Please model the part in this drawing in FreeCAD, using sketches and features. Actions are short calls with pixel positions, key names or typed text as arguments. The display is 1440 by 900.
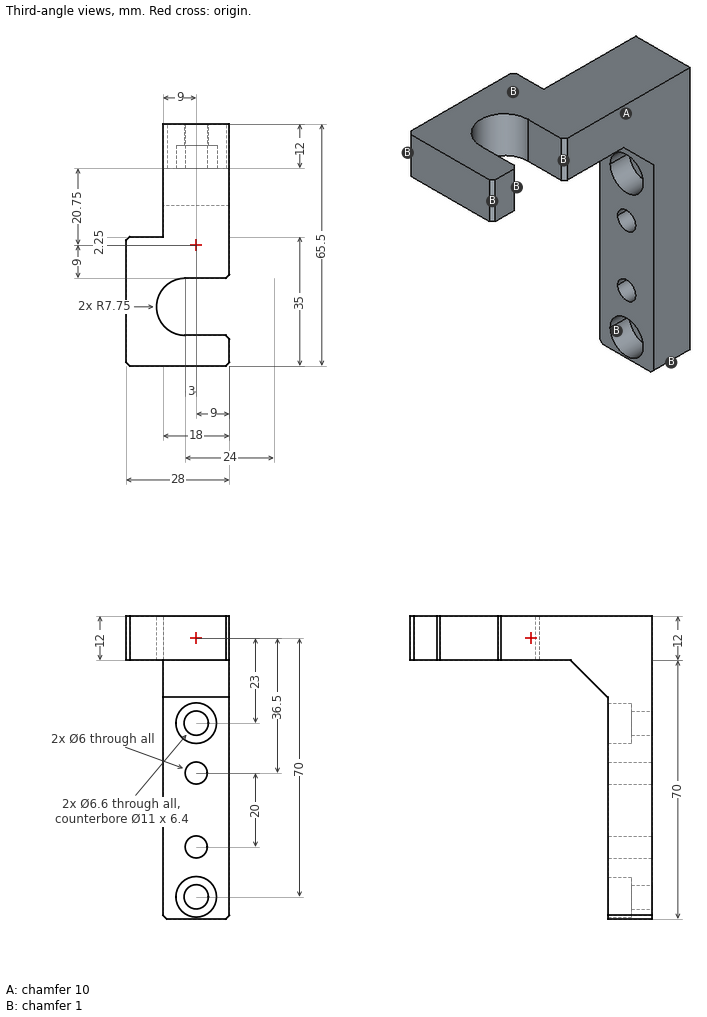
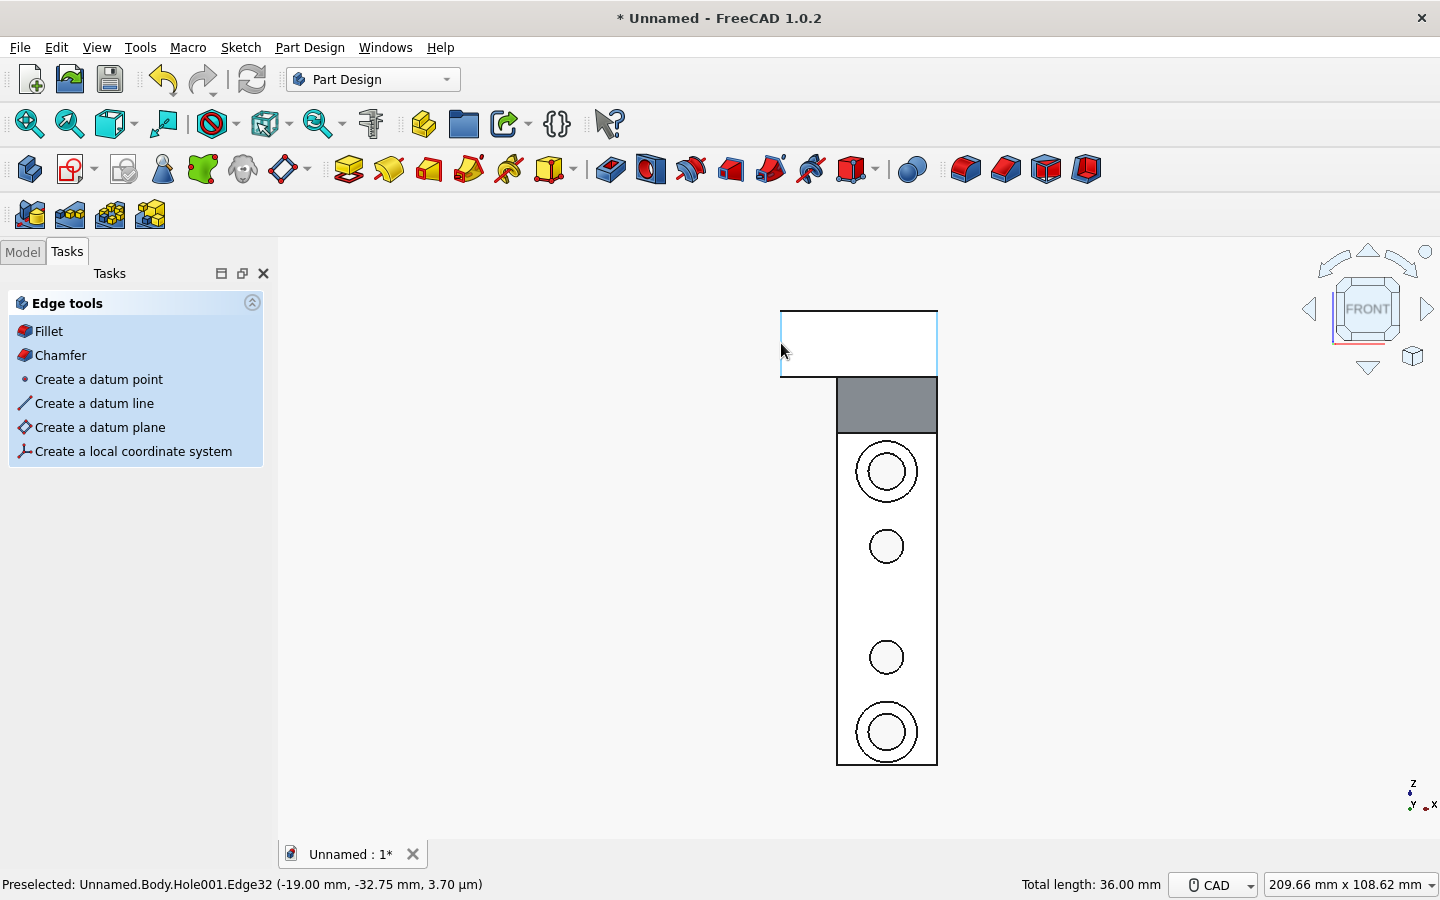
key(3)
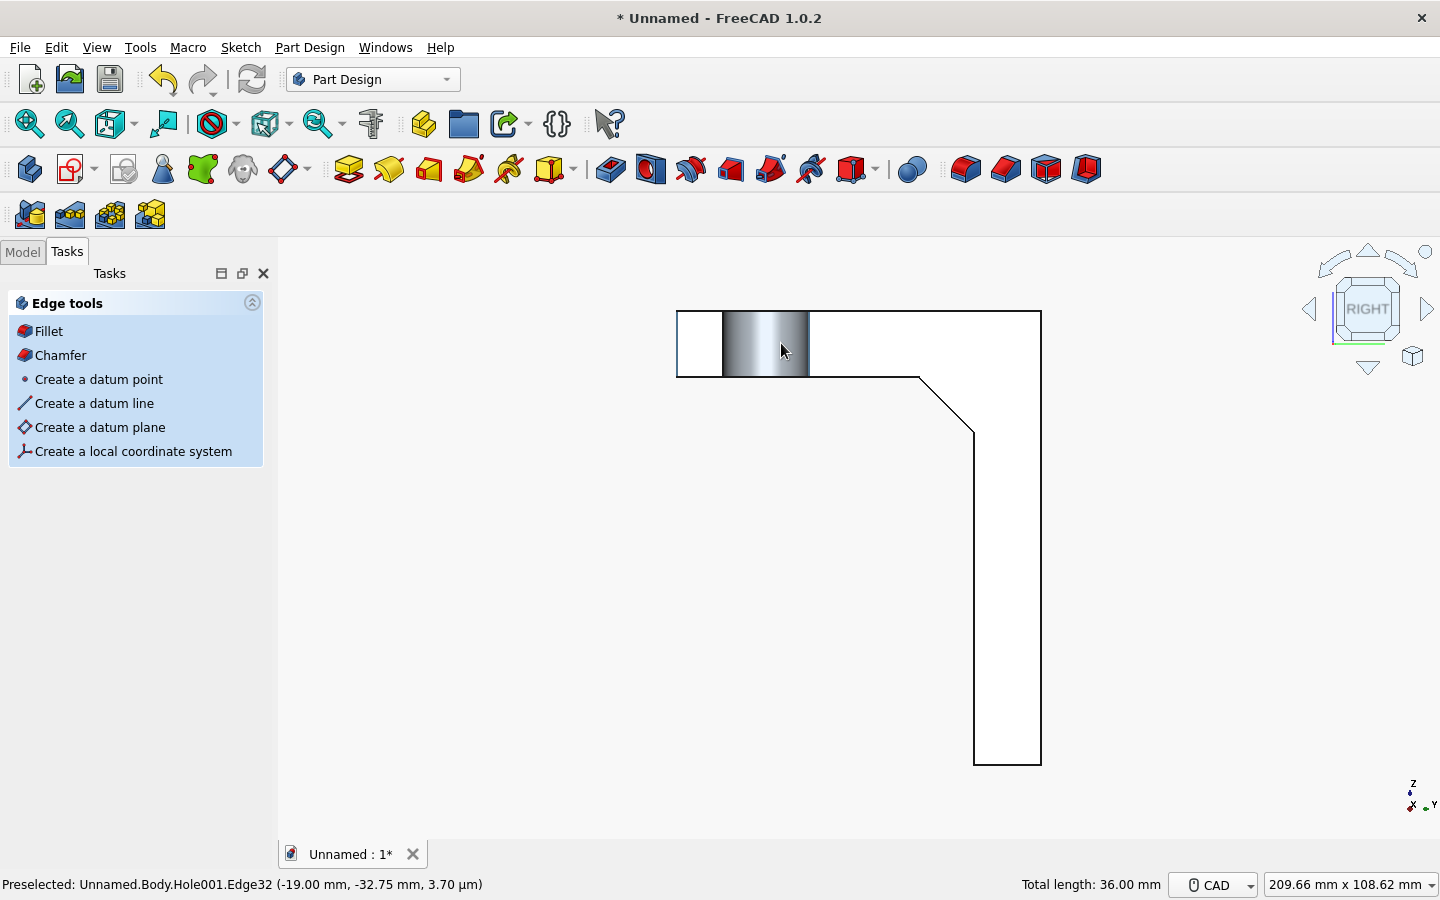
click(723, 343, ctrl)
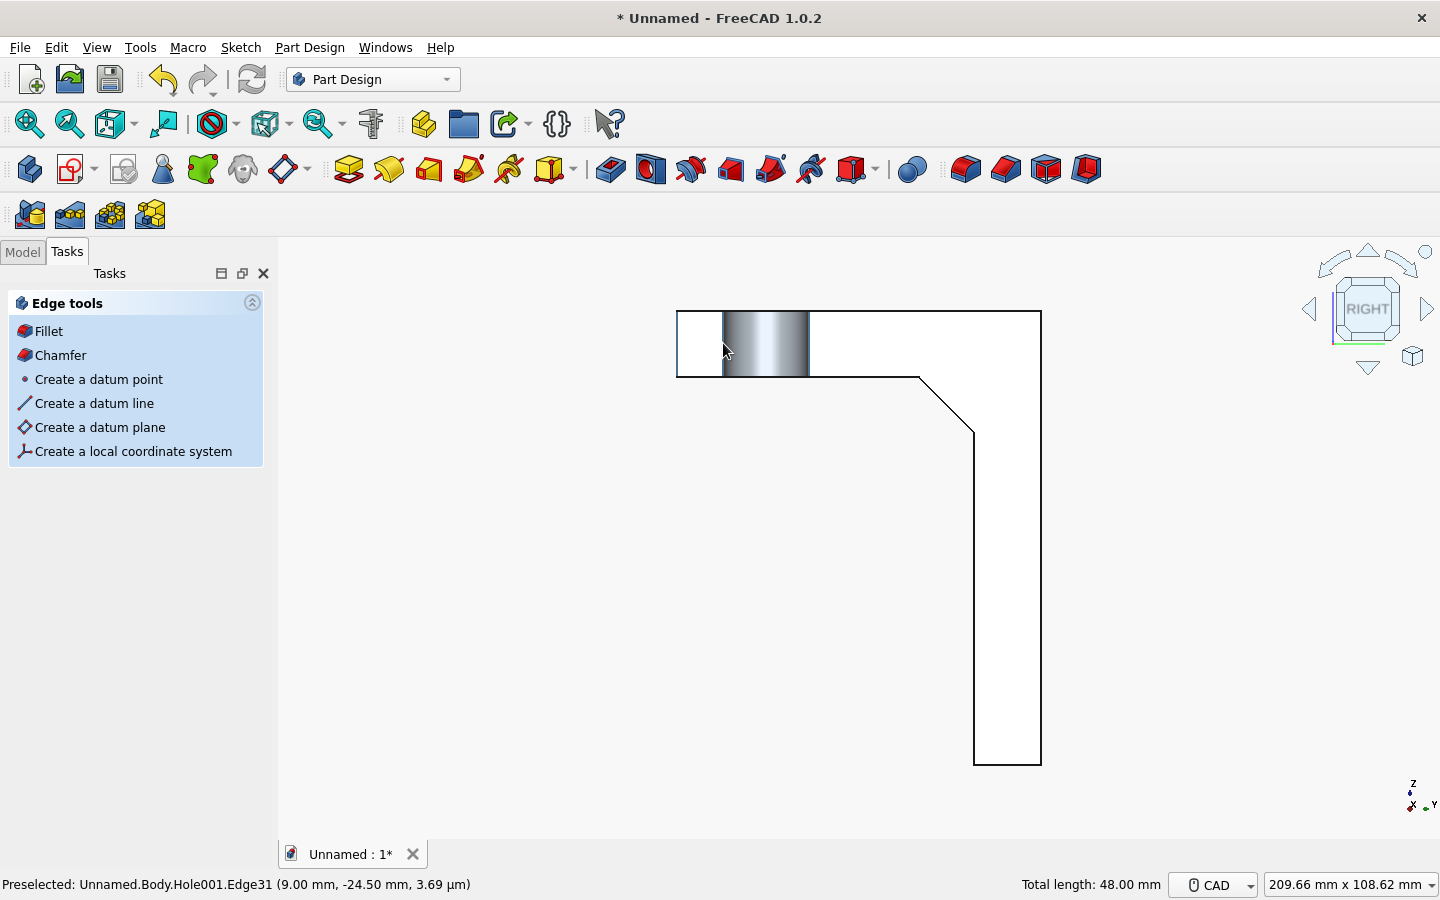
click(1007, 764, ctrl)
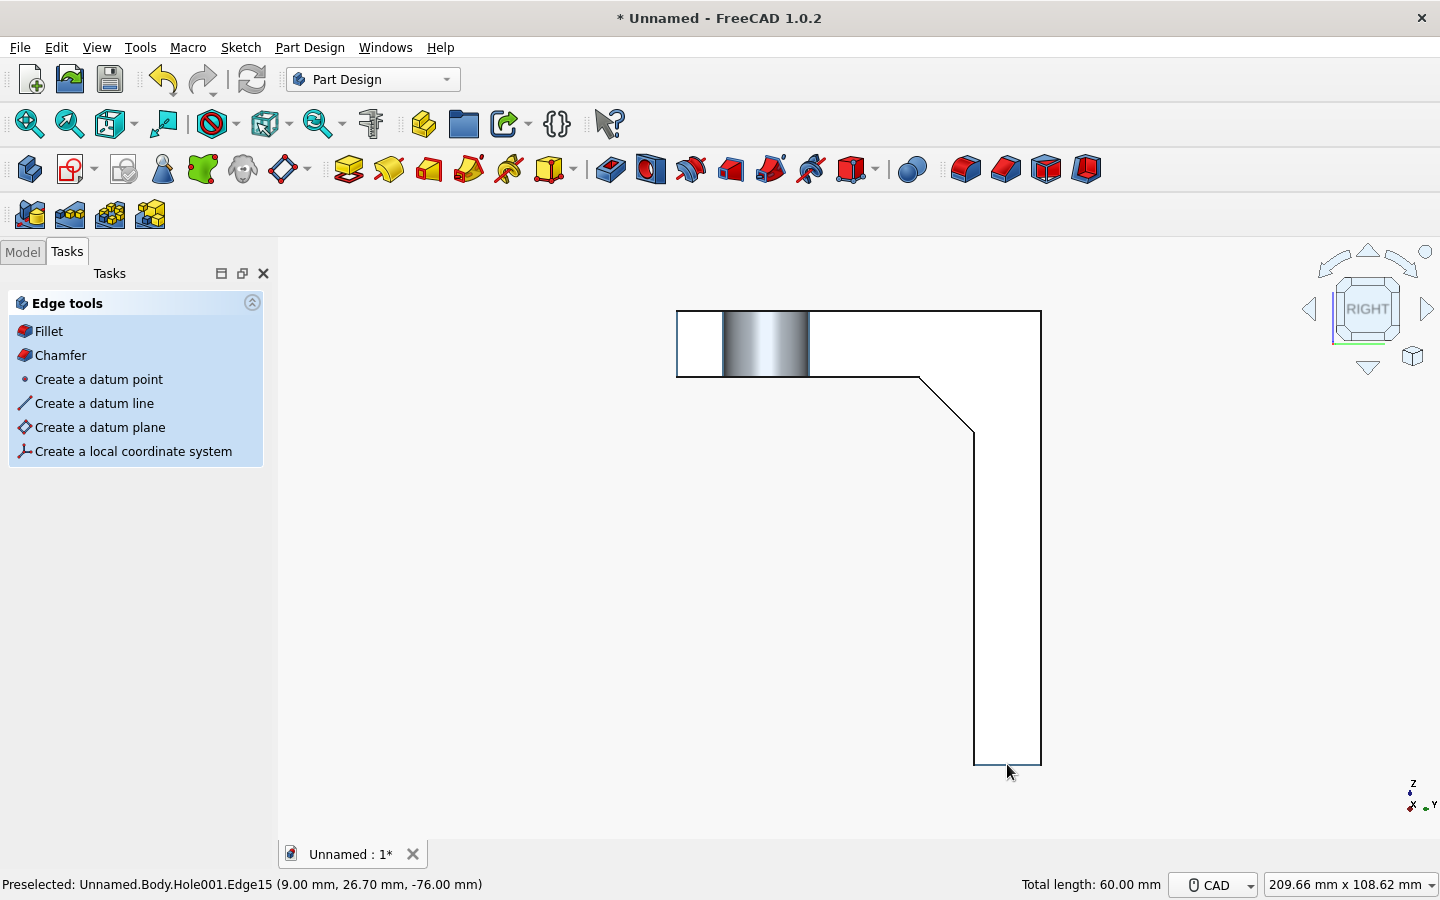
key(5)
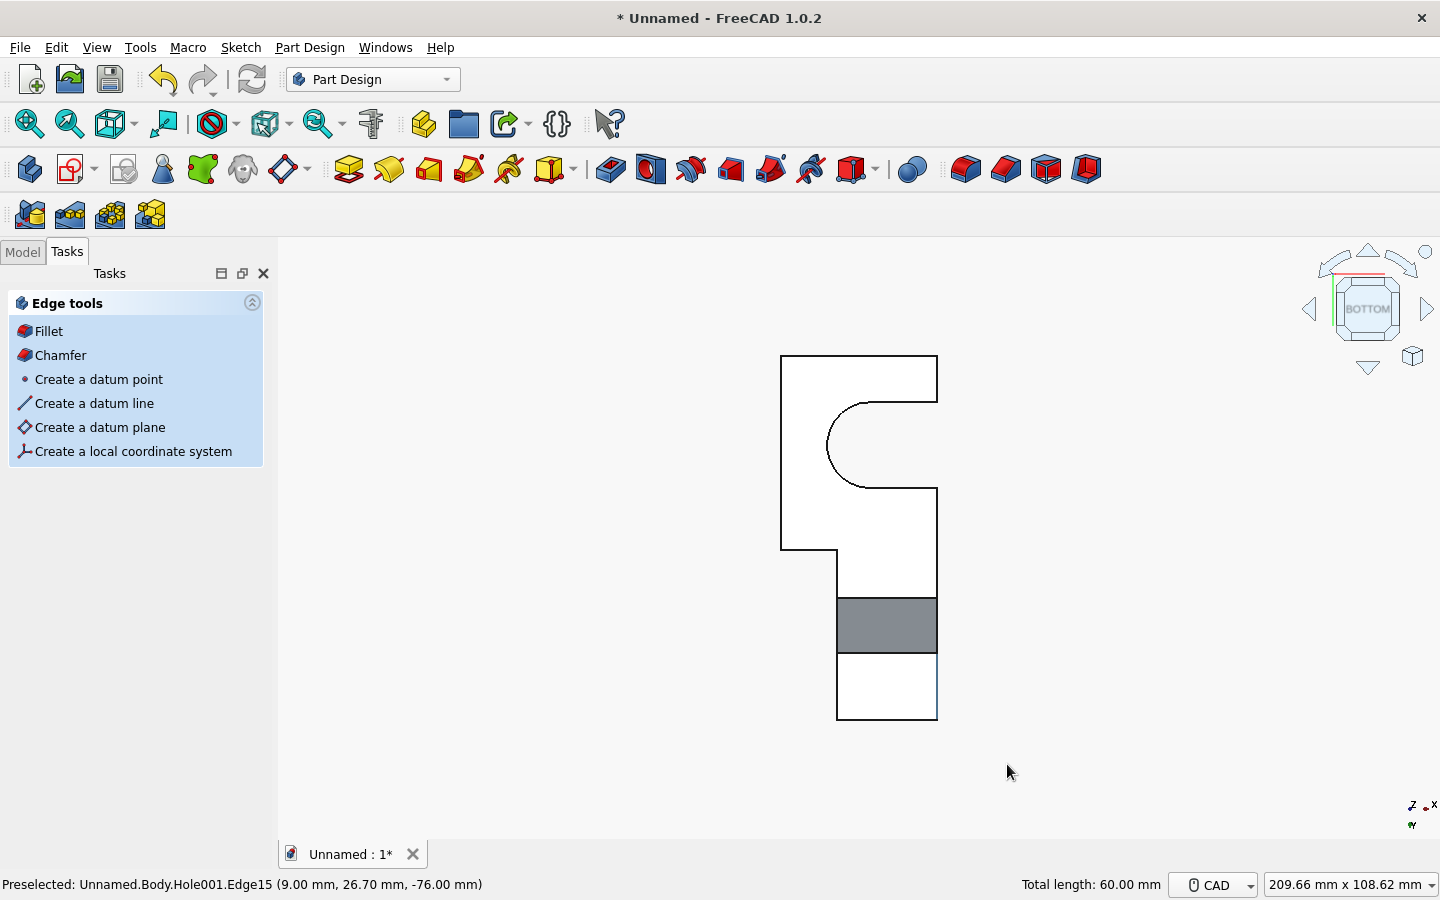
click(837, 685, ctrl)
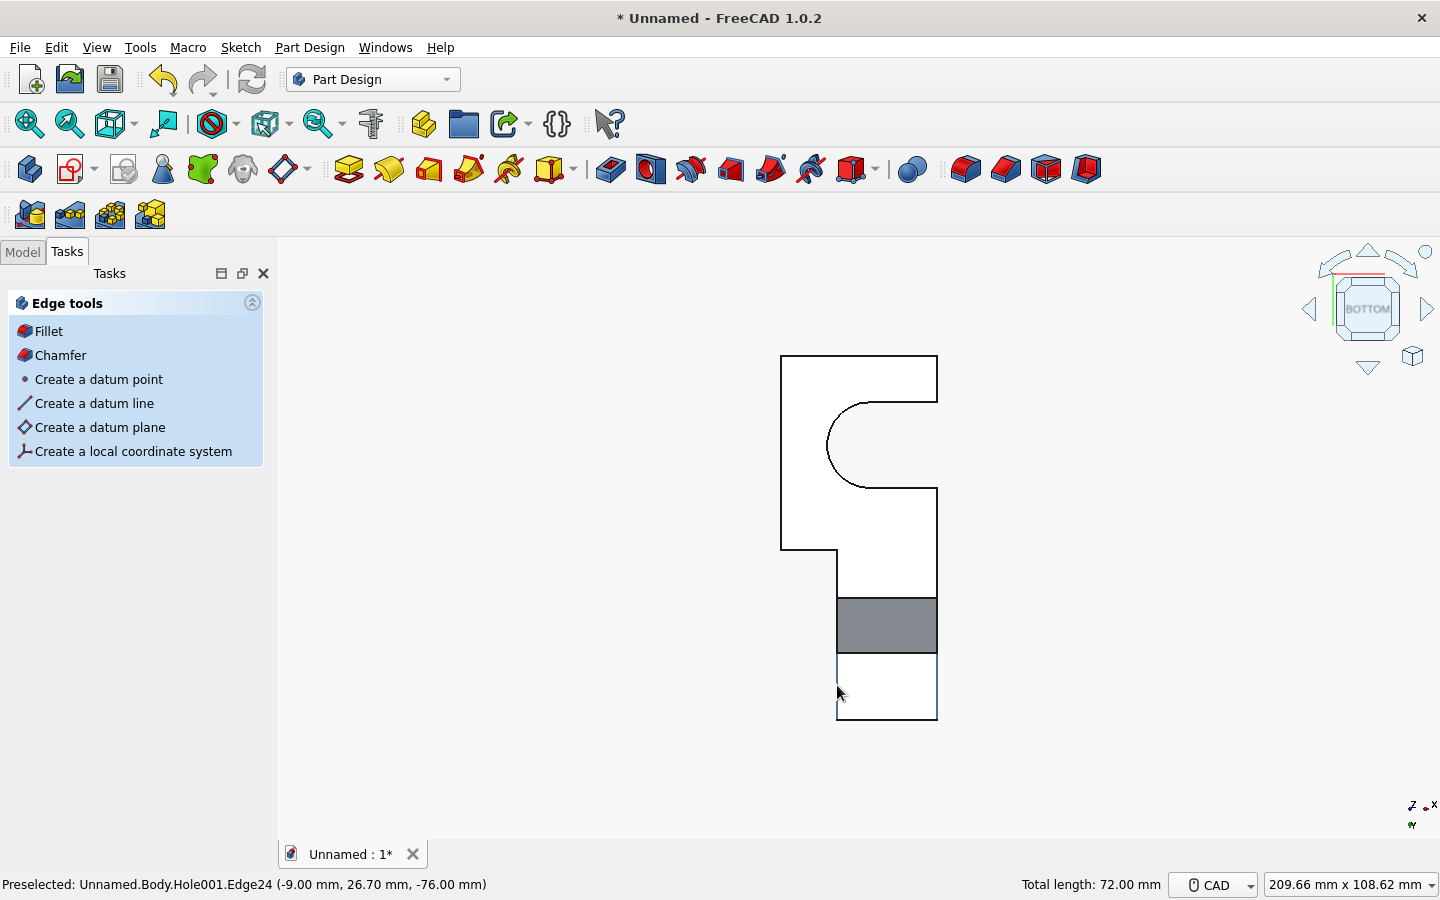
key(4)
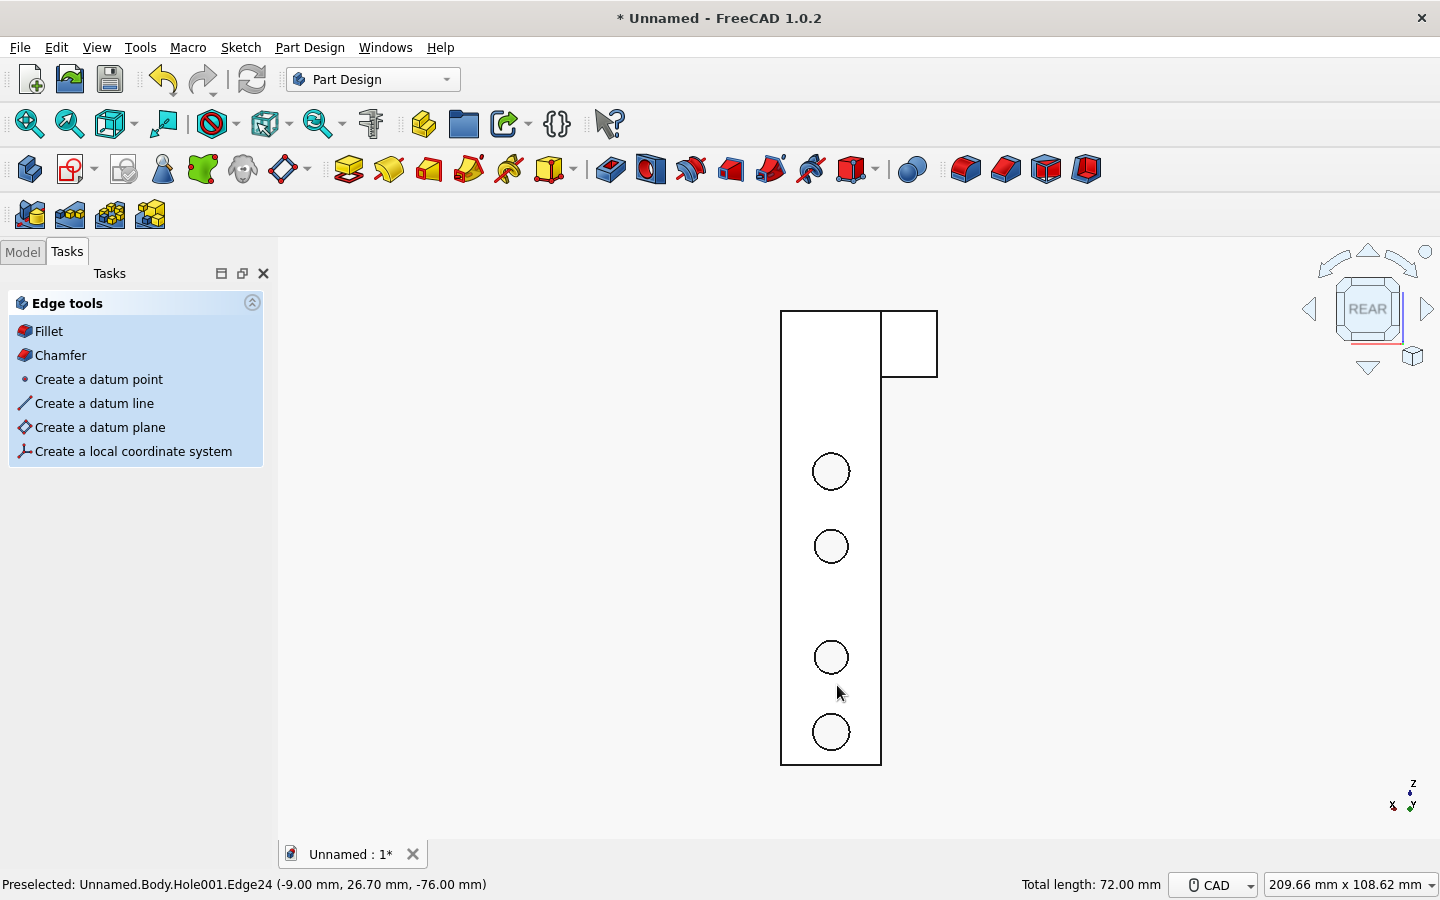
click(937, 343, ctrl)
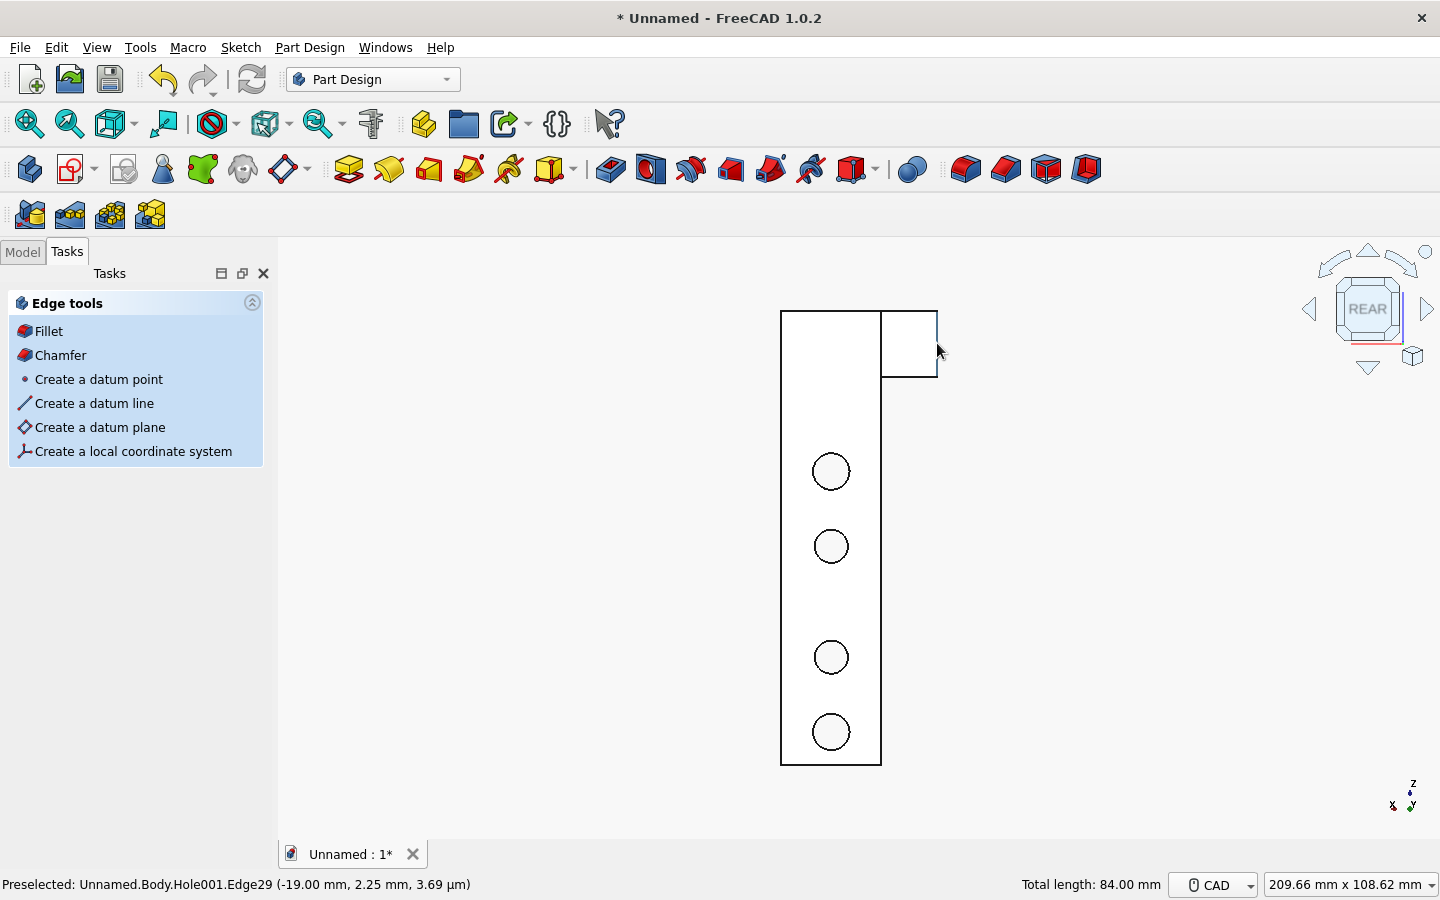
click(1006, 170)